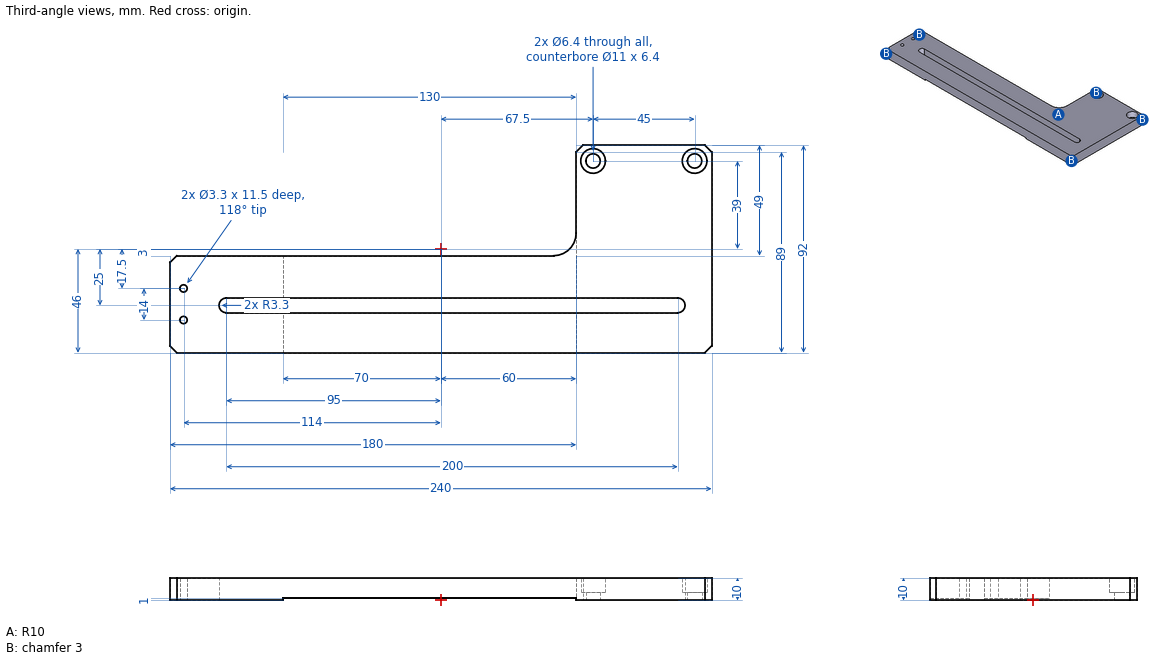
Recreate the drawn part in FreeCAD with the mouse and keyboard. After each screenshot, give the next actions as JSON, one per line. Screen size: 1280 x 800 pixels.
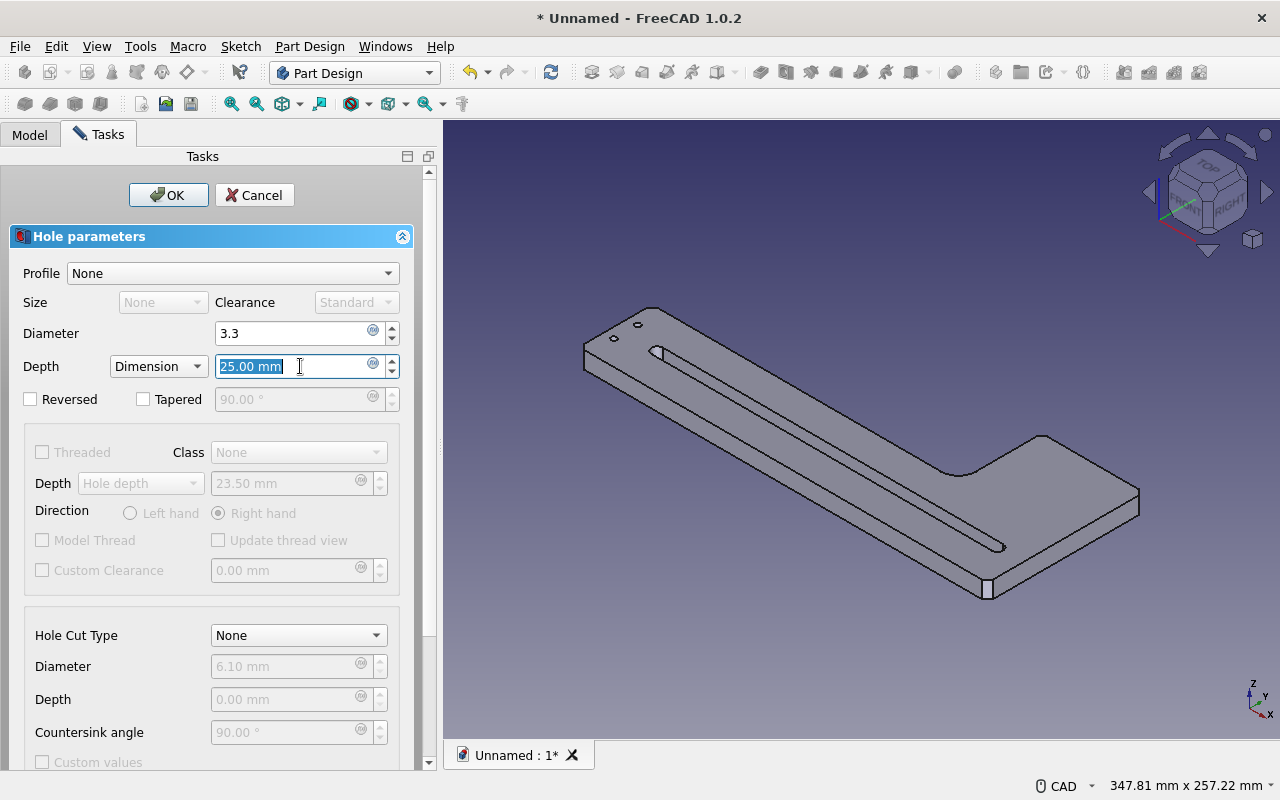
{"action": "type", "text": "11.5"}
{"action": "key", "text": "Tab"}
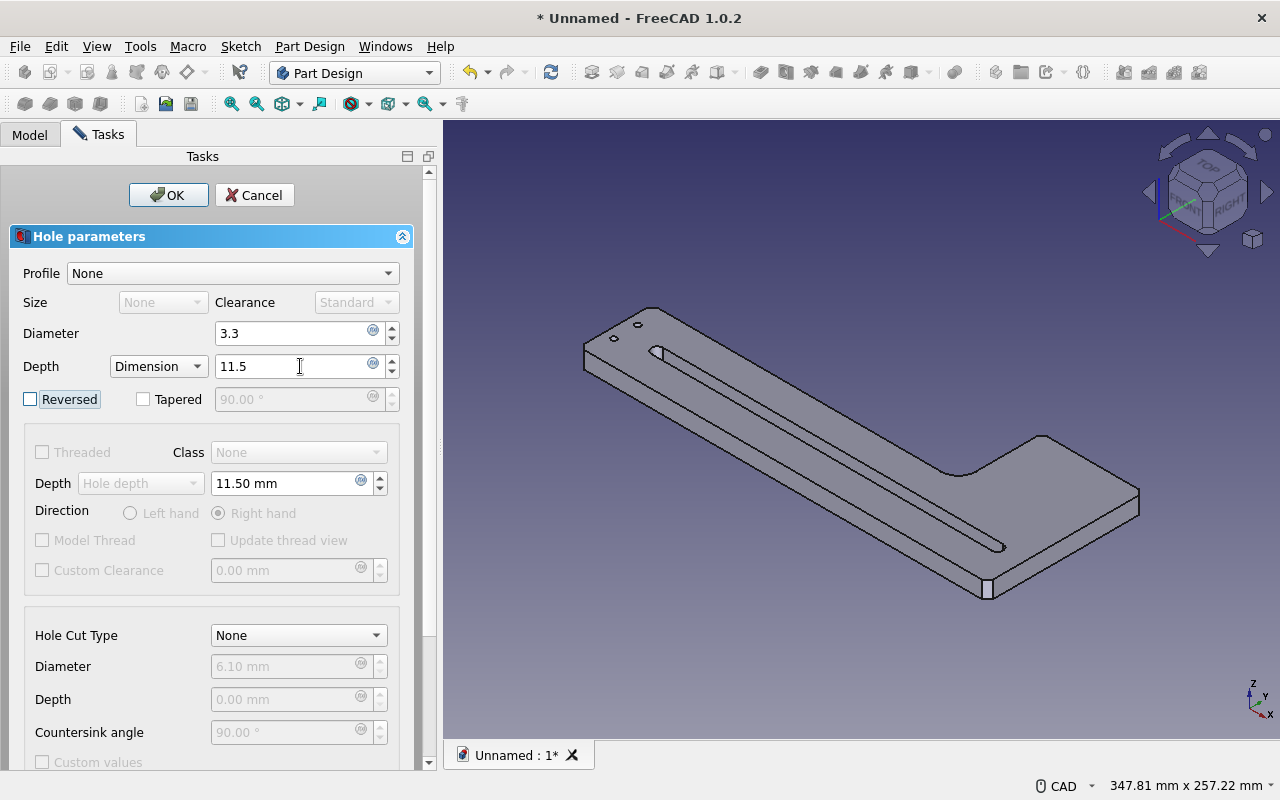
{"action": "left_click", "coordinate": [169, 195]}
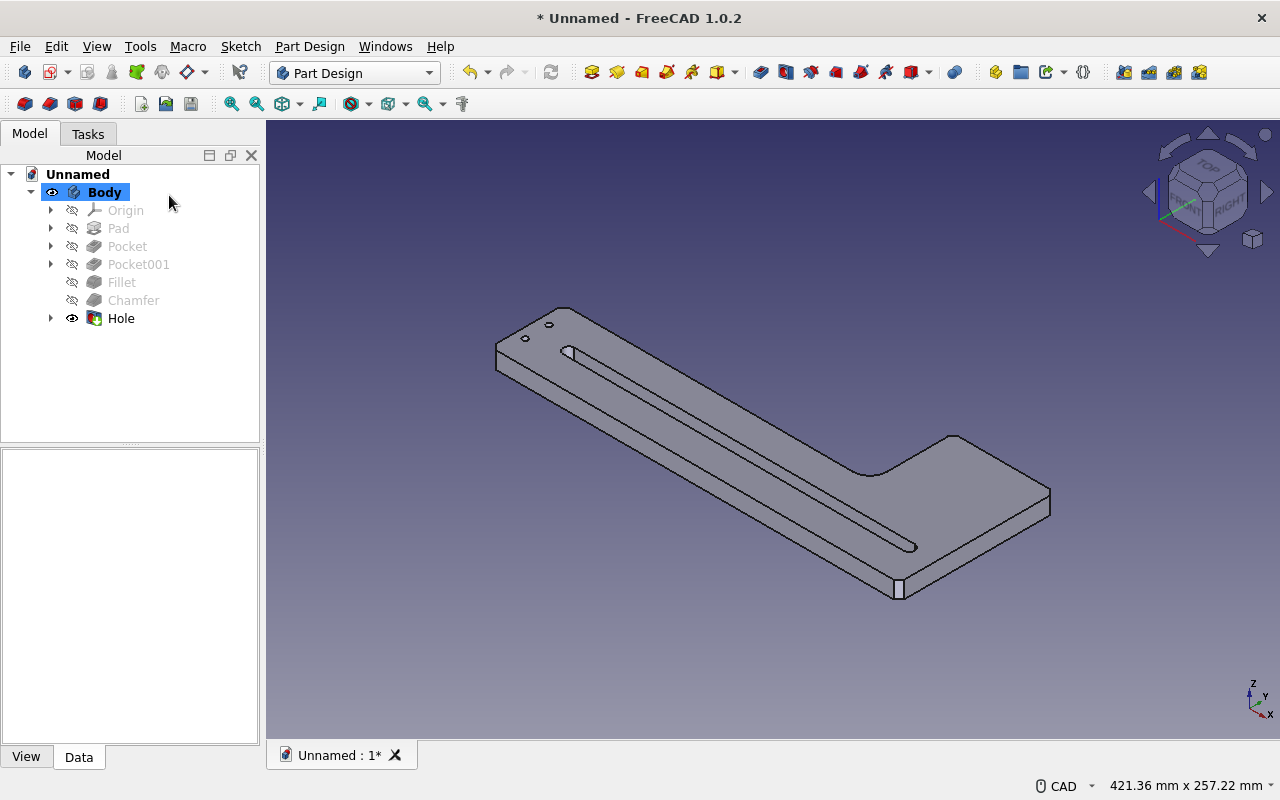
{"action": "left_click", "coordinate": [993, 494]}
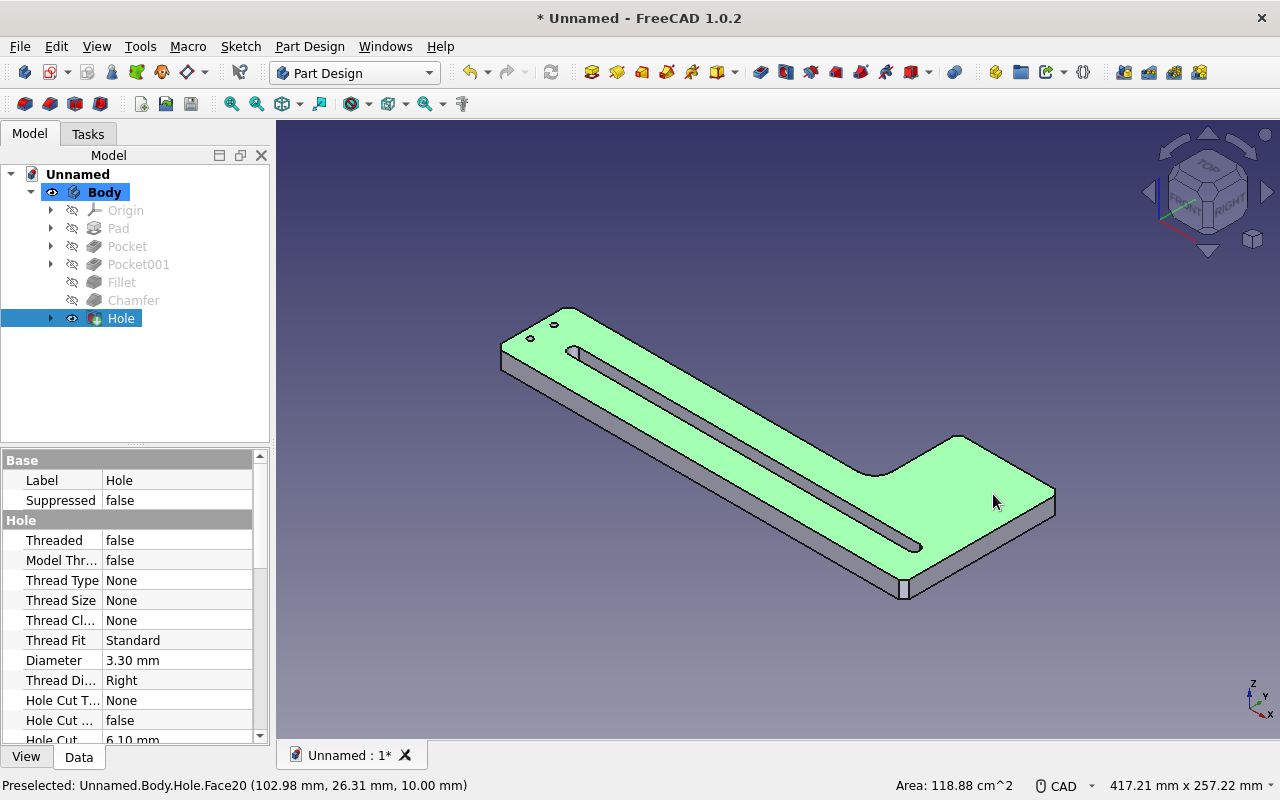
{"action": "left_click", "coordinate": [50, 72]}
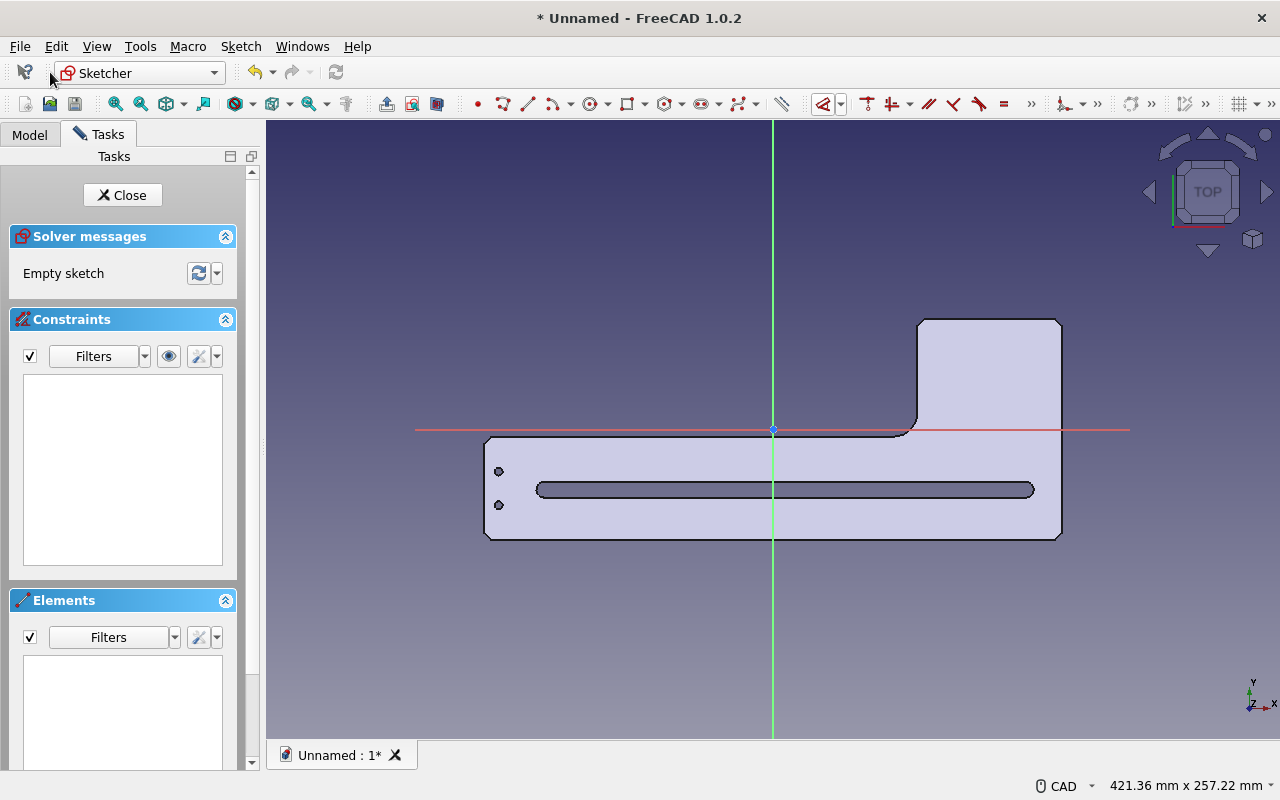
{"action": "scroll", "coordinate": [1082, 337], "scroll_direction": "up", "scroll_amount": 4}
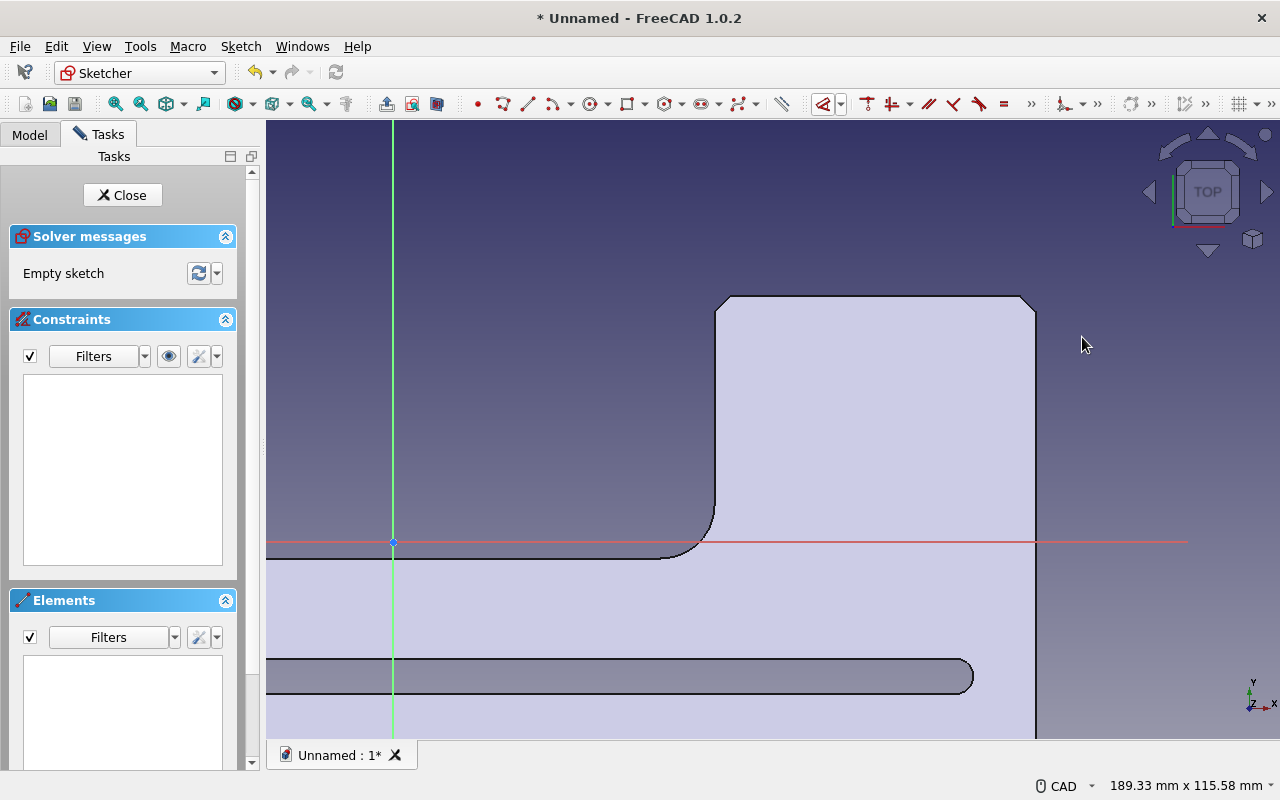
{"action": "key", "text": "g c"}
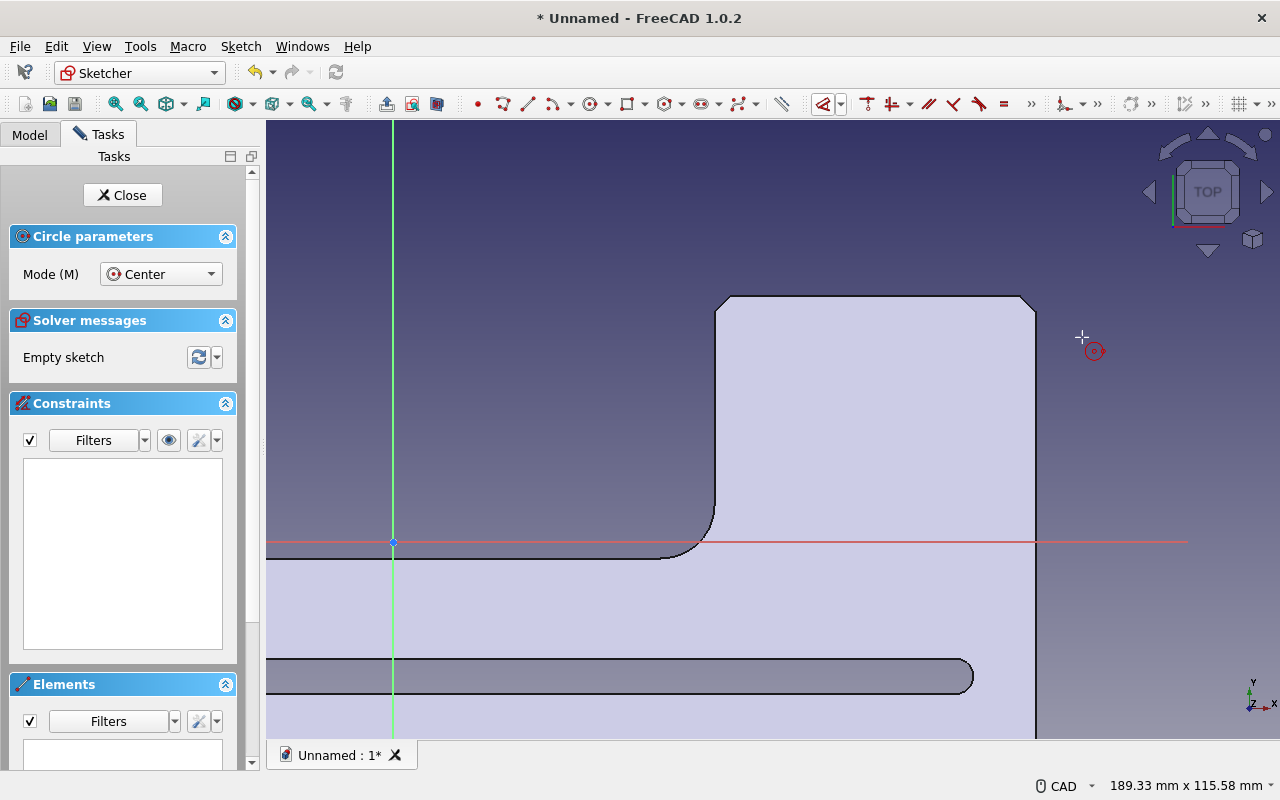
{"action": "scroll", "coordinate": [755, 334], "scroll_direction": "up", "scroll_amount": 2}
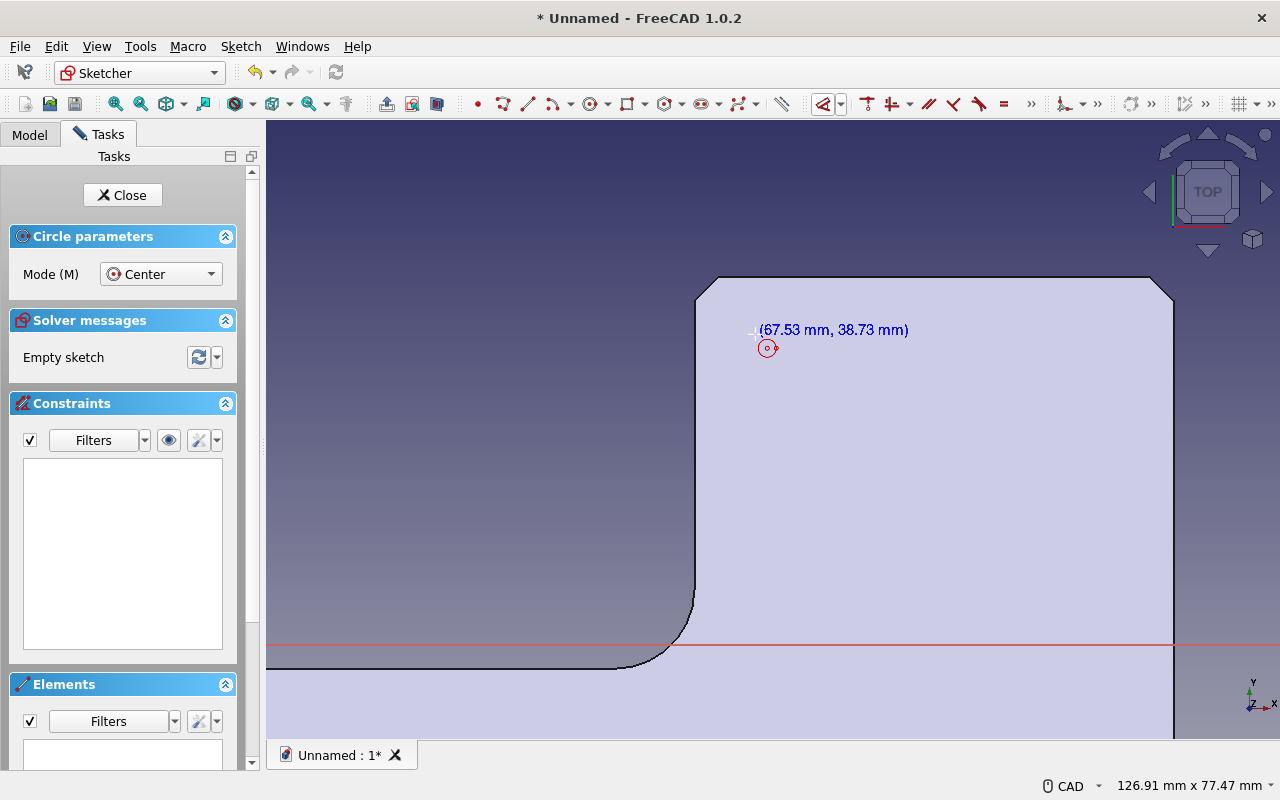
{"action": "left_click", "coordinate": [755, 333]}
{"action": "mouse_move", "coordinate": [773, 315]}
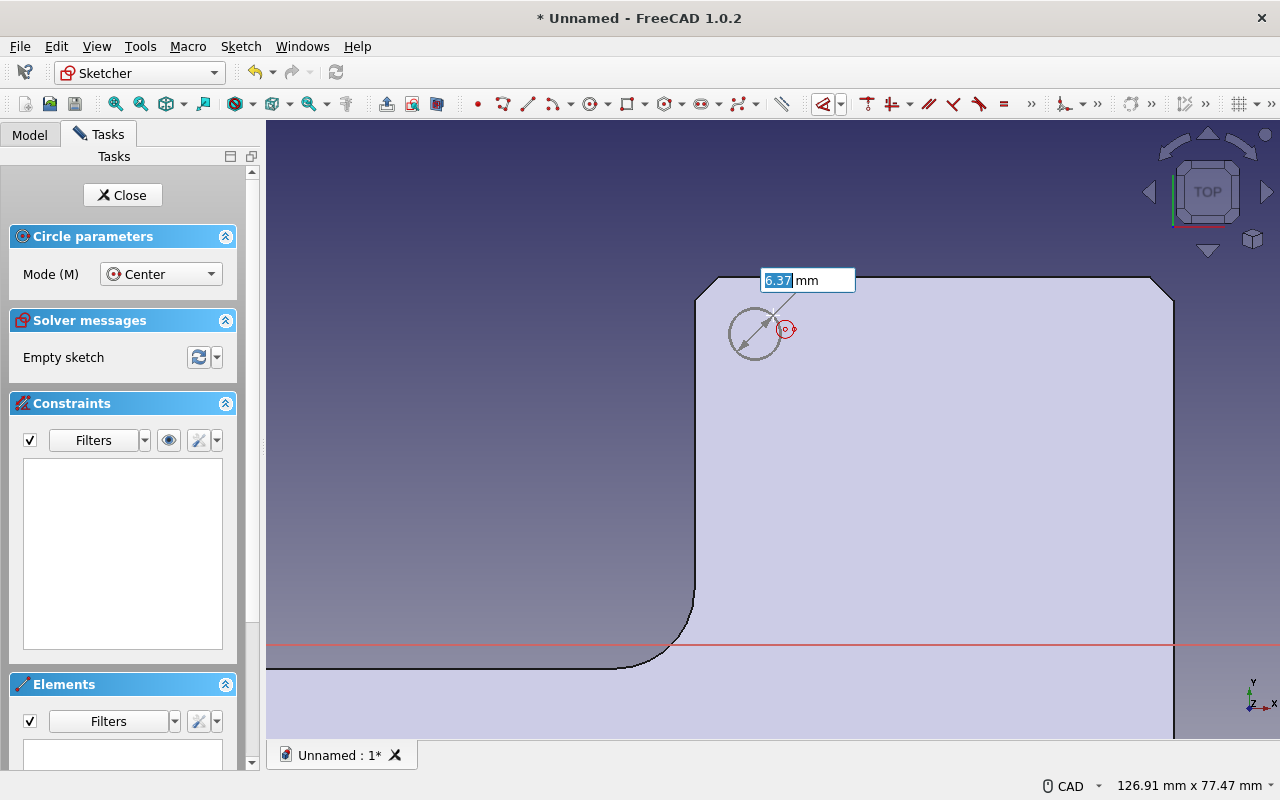
{"action": "type", "text": "6.4"}
{"action": "key", "text": "Return"}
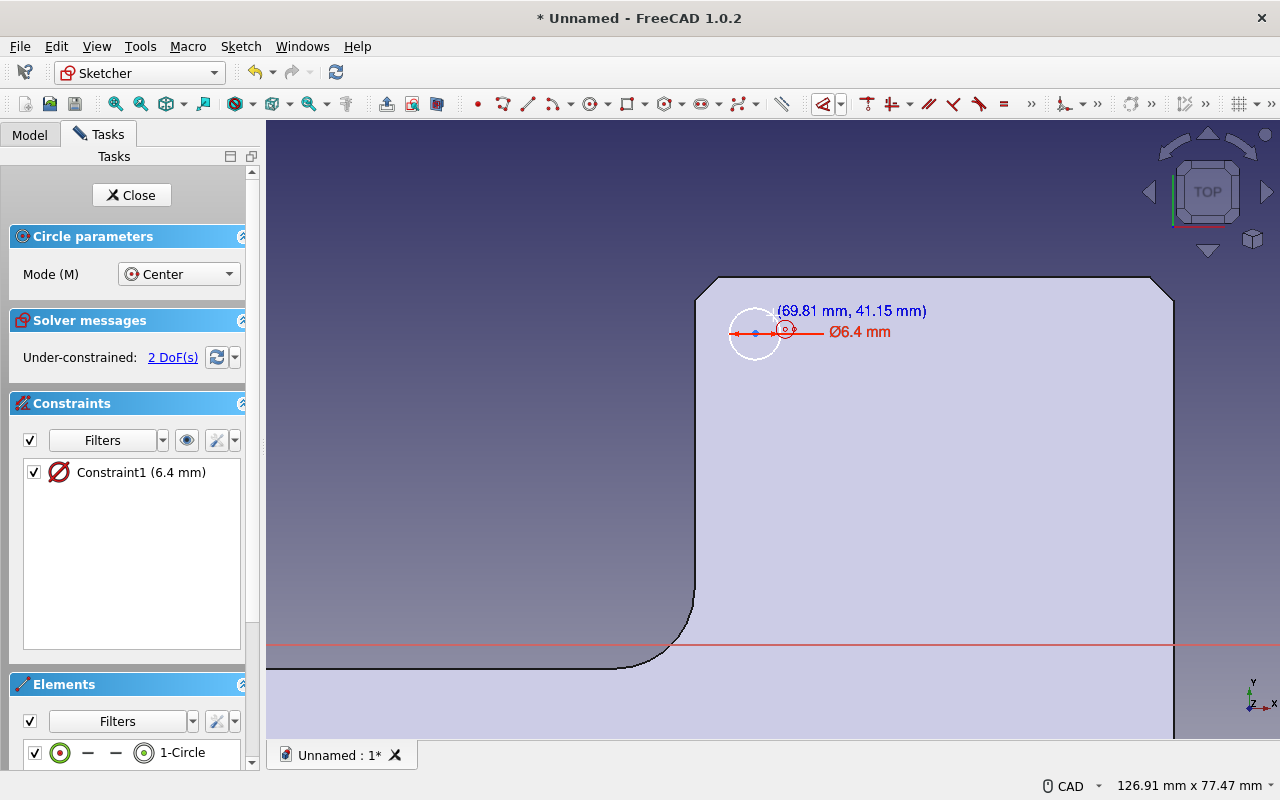
{"action": "left_click", "coordinate": [1114, 333]}